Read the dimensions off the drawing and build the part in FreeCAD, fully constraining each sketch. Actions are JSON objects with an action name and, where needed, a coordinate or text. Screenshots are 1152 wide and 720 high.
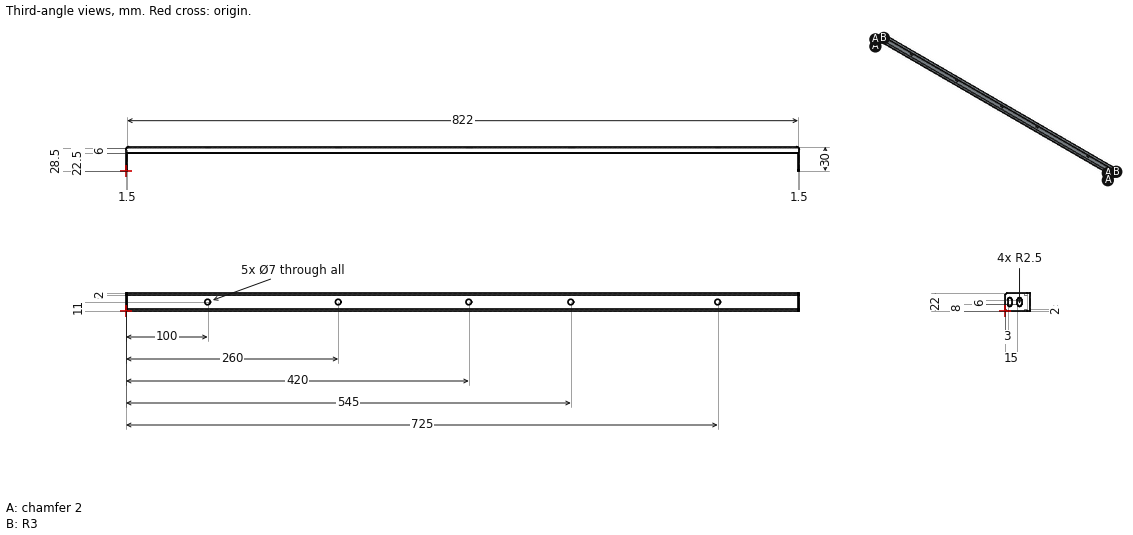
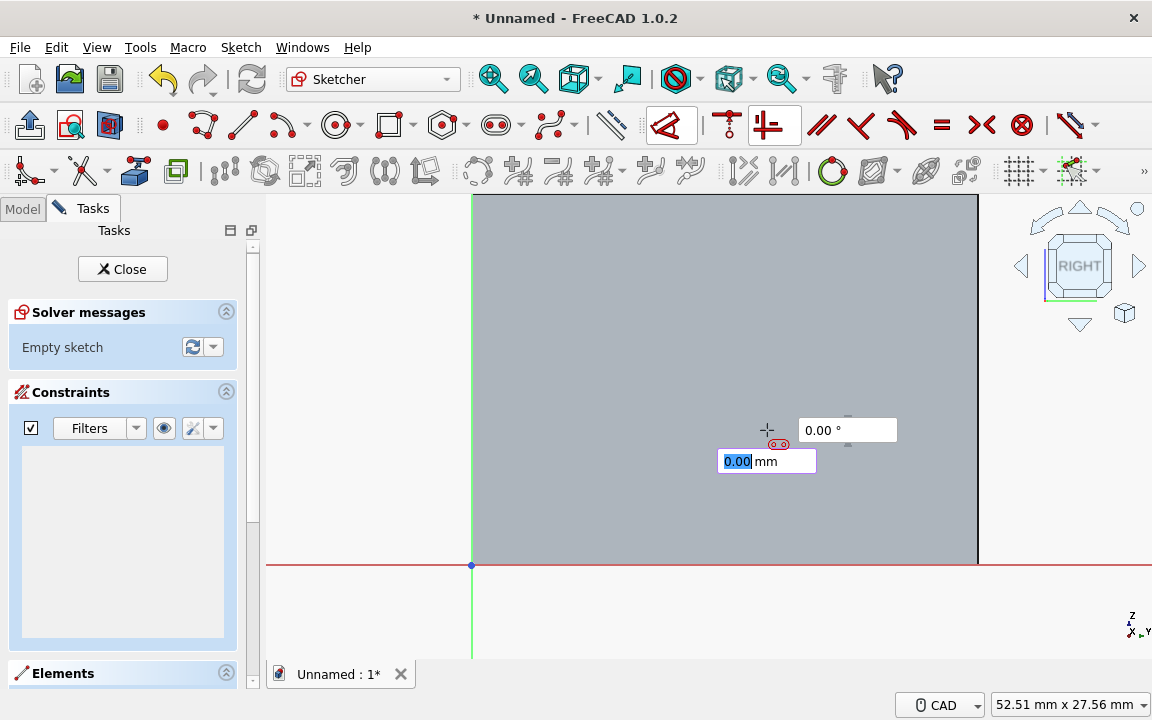
{"action": "left_click", "coordinate": [767, 329]}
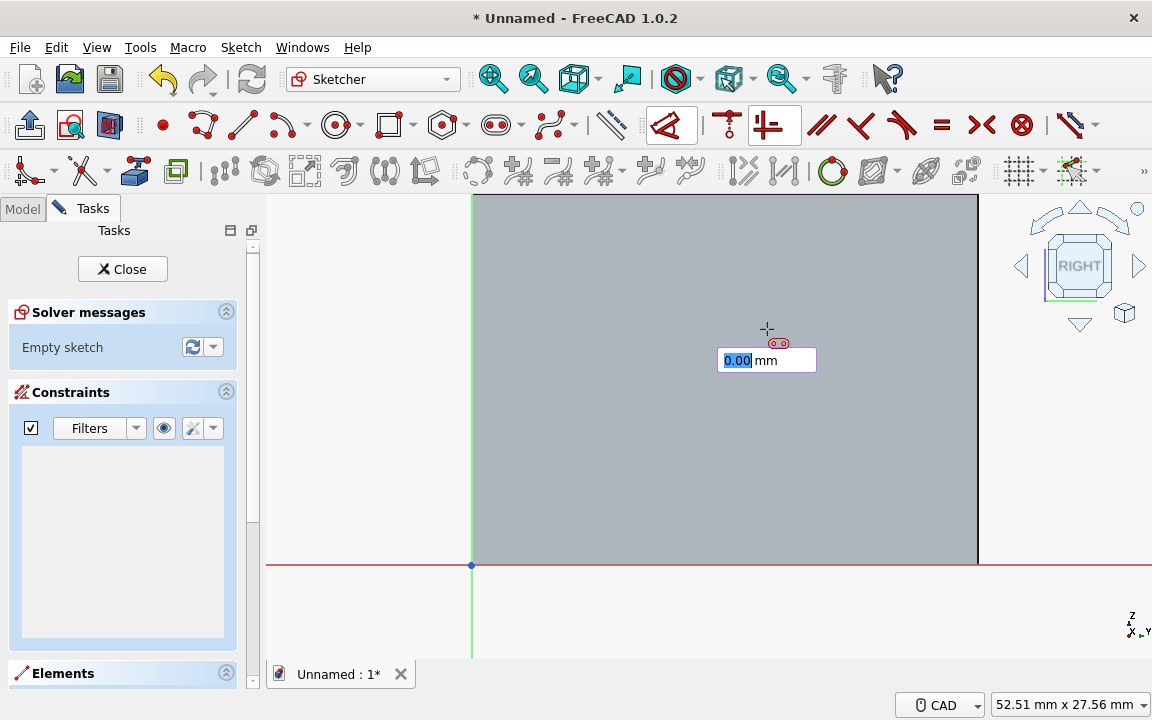
{"action": "left_click", "coordinate": [809, 380]}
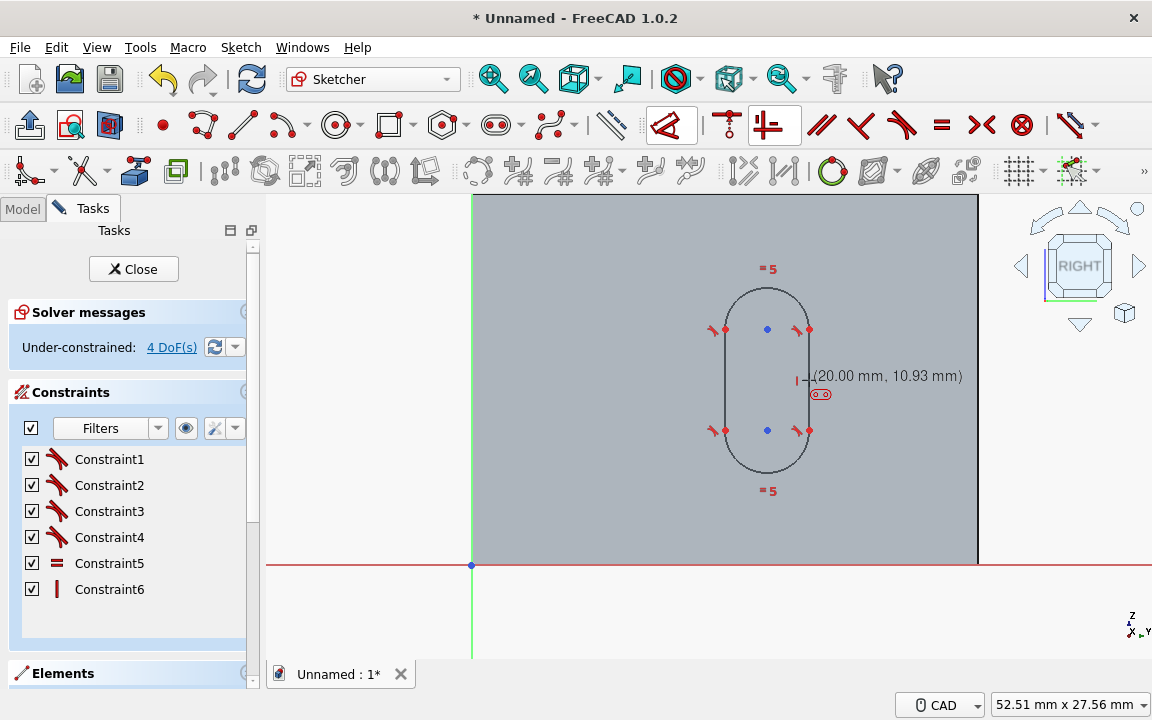
{"action": "left_click", "coordinate": [564, 430]}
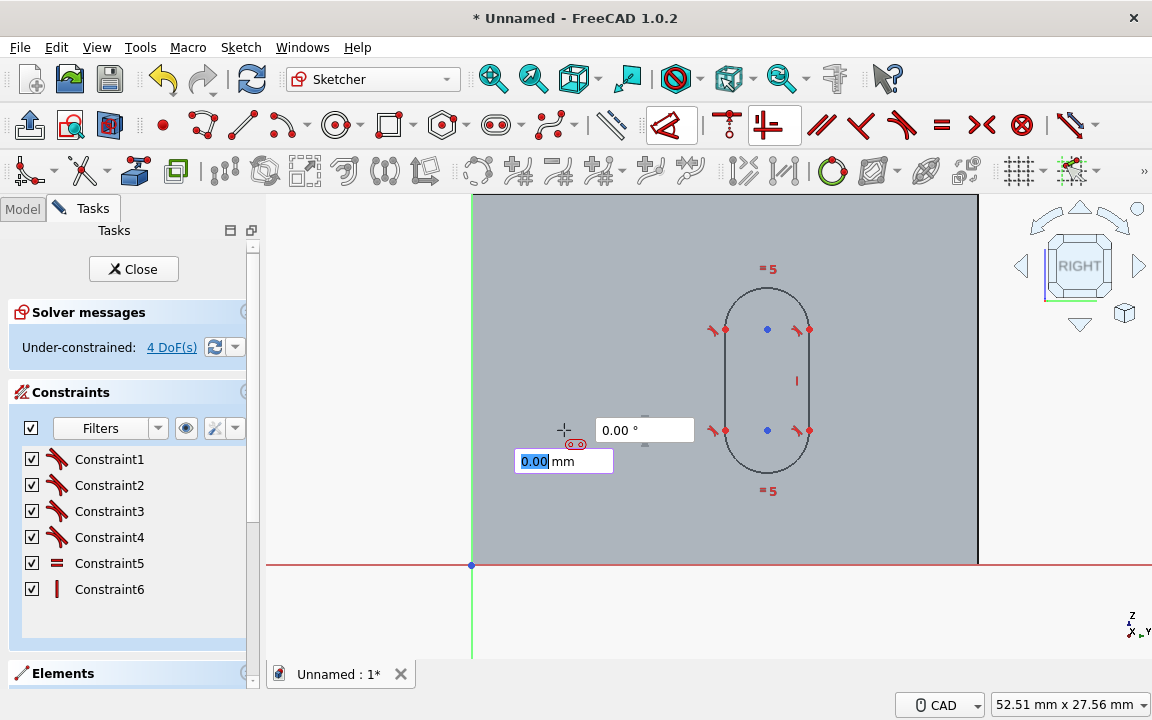
{"action": "left_click", "coordinate": [564, 329]}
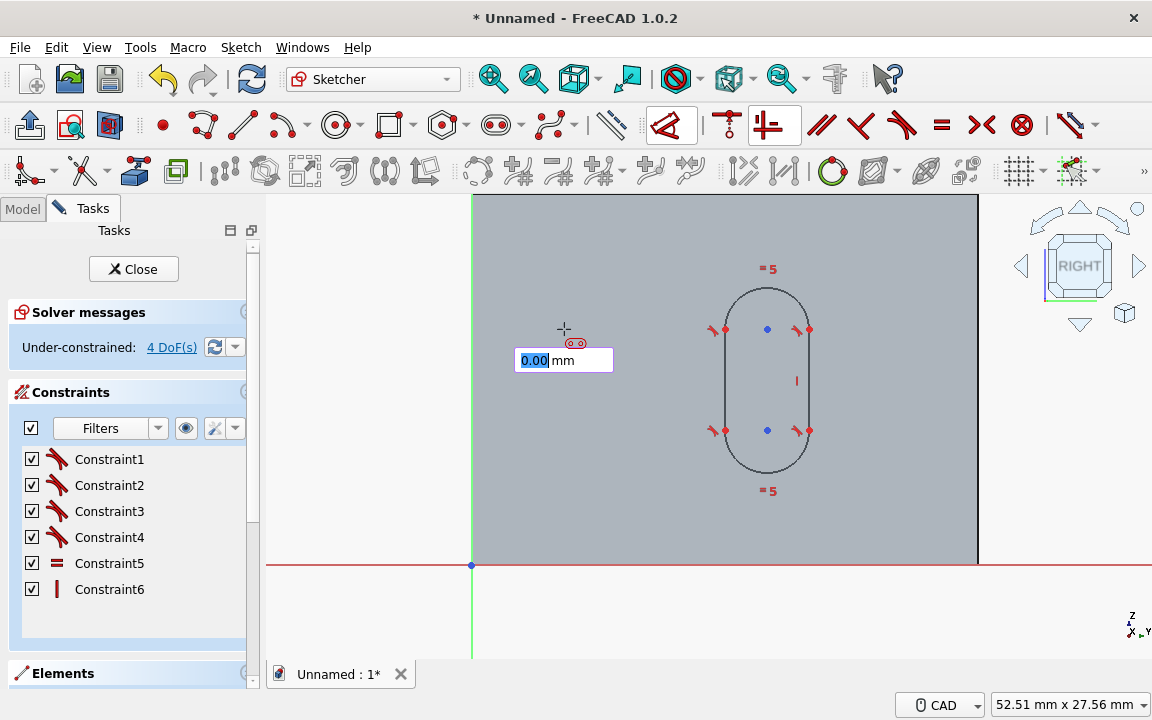
{"action": "left_click", "coordinate": [606, 380]}
{"action": "key", "text": "Escape"}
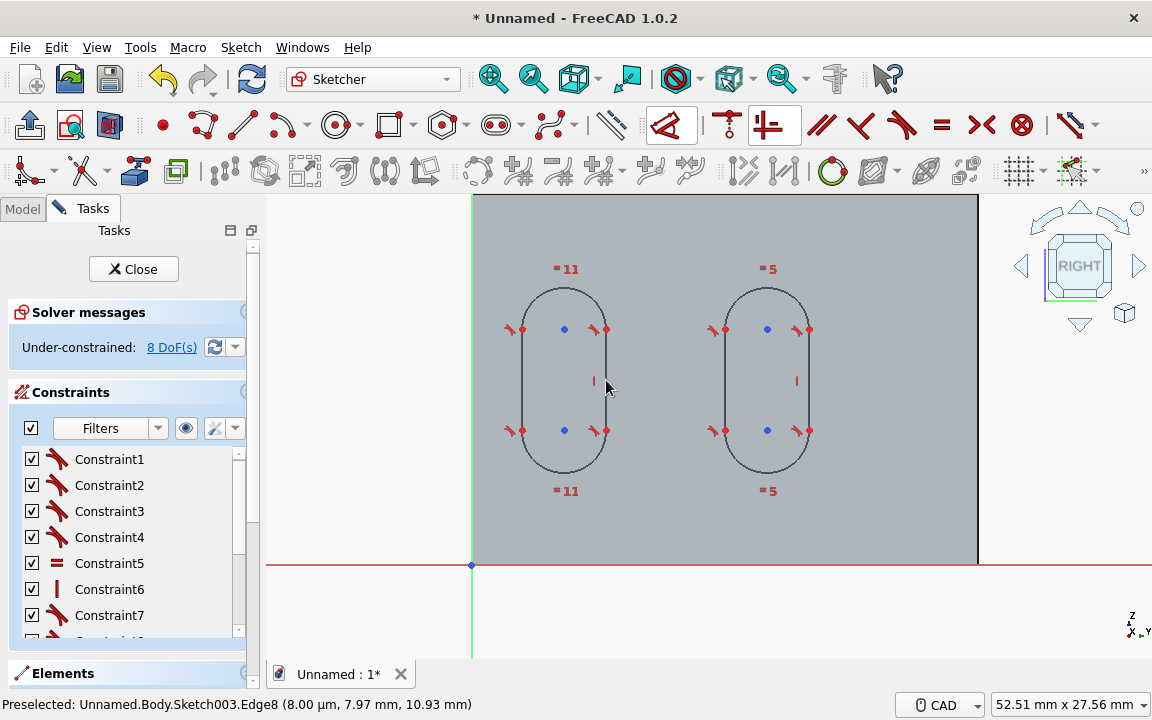
{"action": "left_click", "coordinate": [742, 465]}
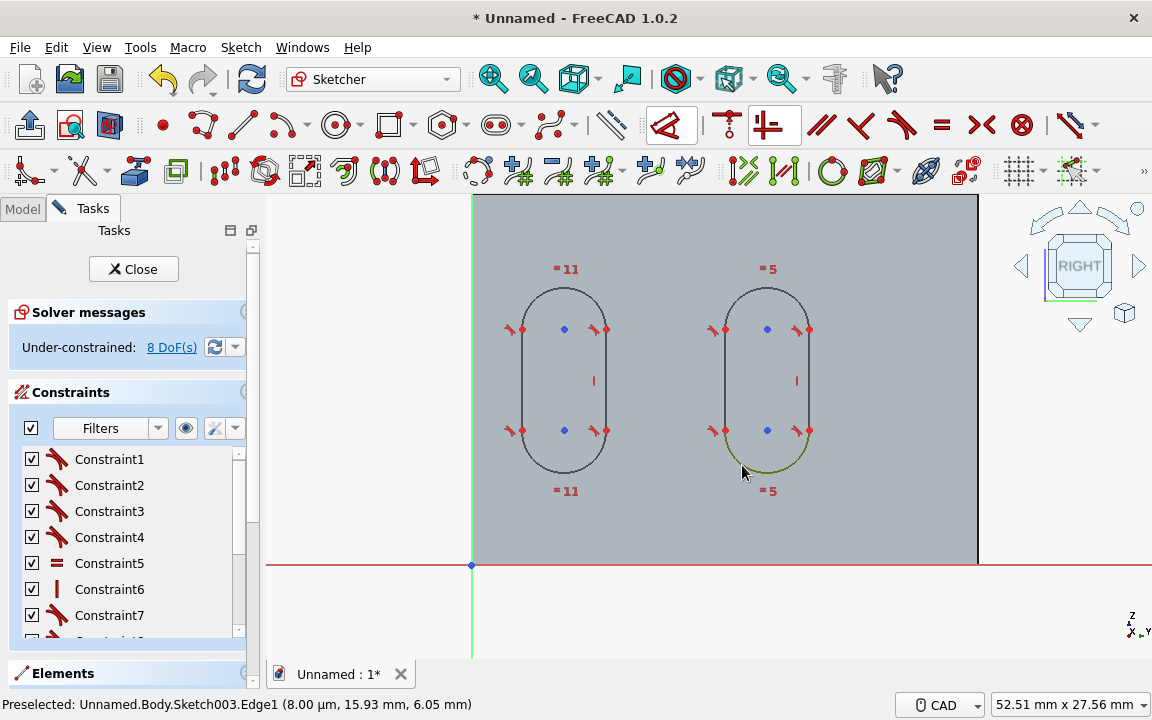
{"action": "left_click", "coordinate": [539, 465]}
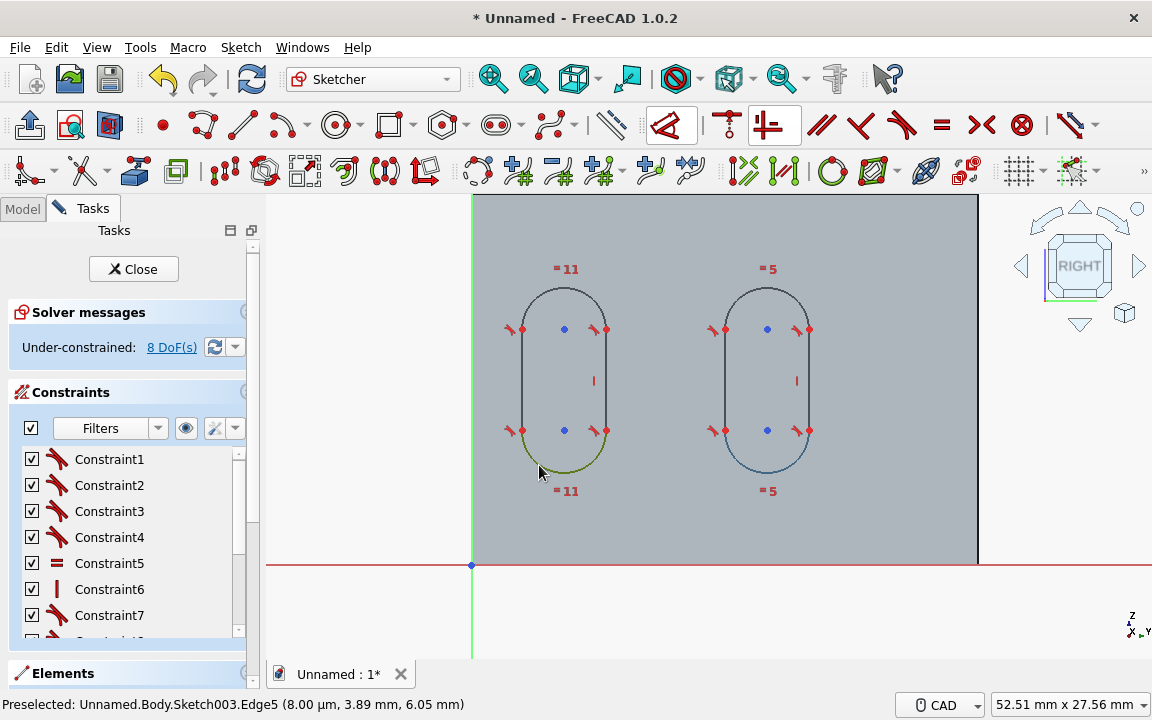
{"action": "left_click", "coordinate": [942, 126]}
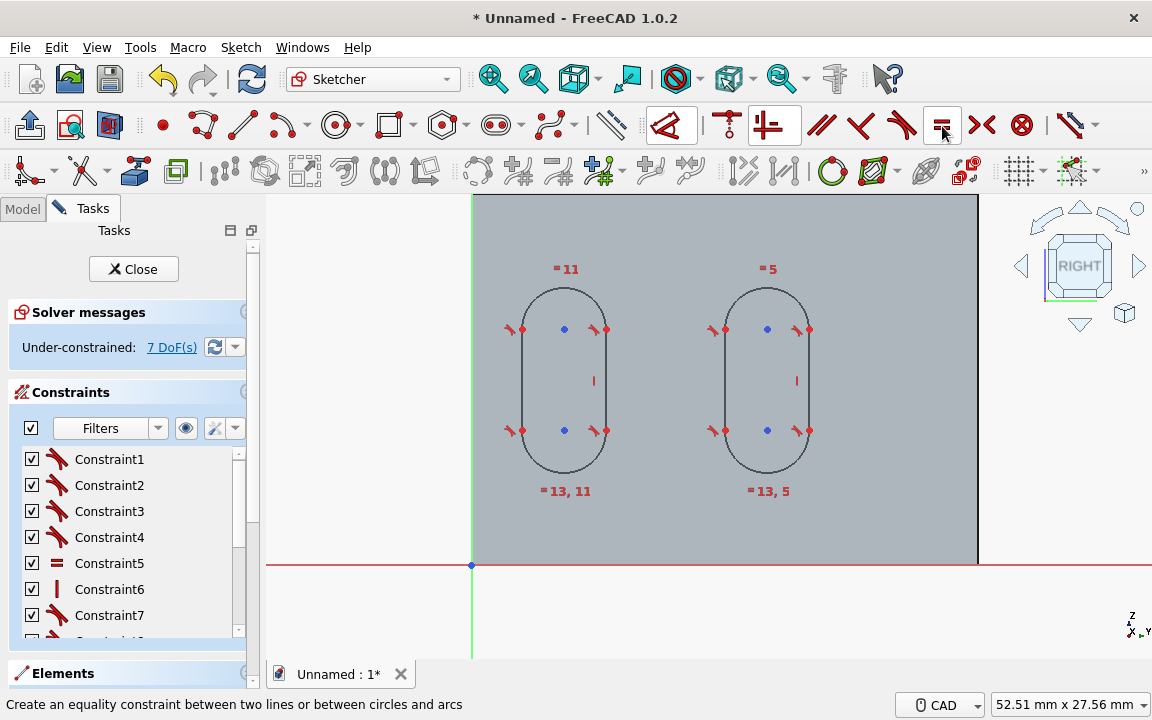
{"action": "left_click", "coordinate": [742, 465]}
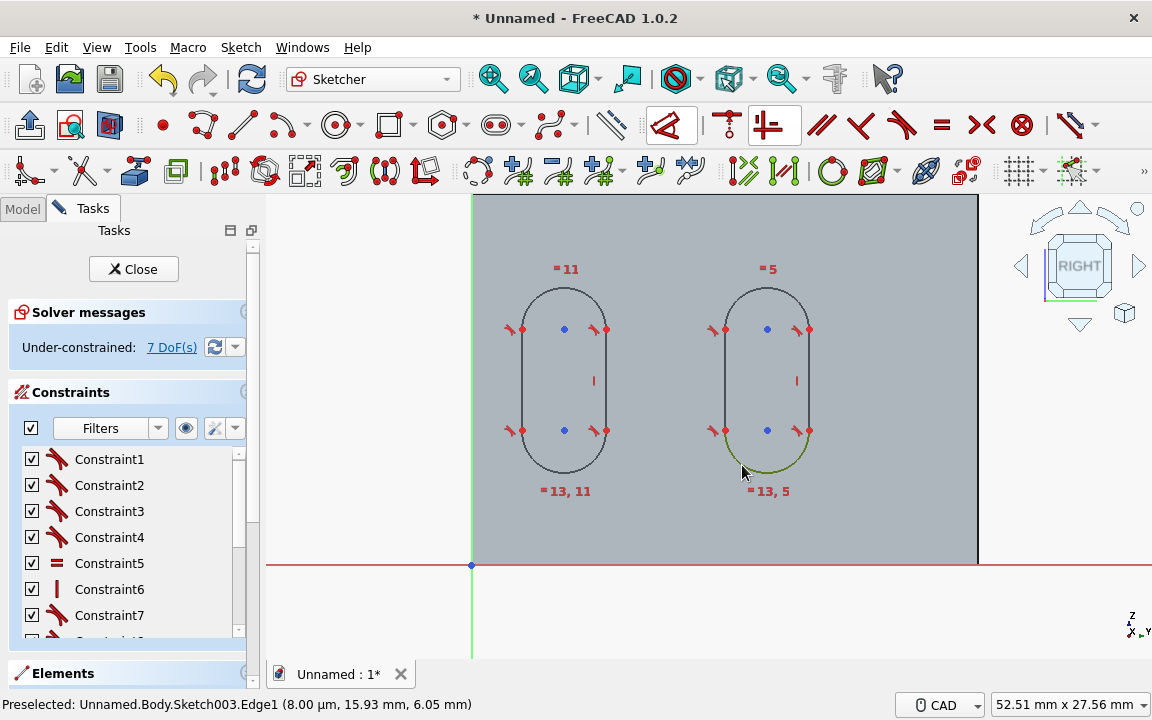
{"action": "left_click", "coordinate": [692, 126]}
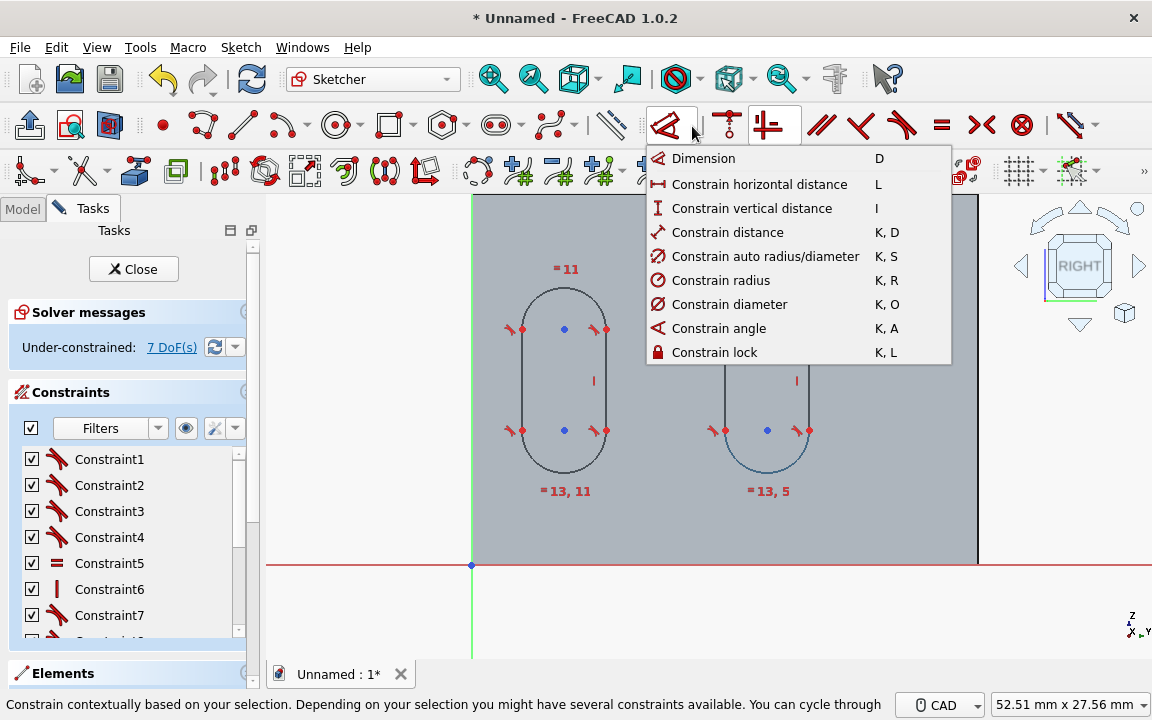
{"action": "left_click", "coordinate": [799, 280]}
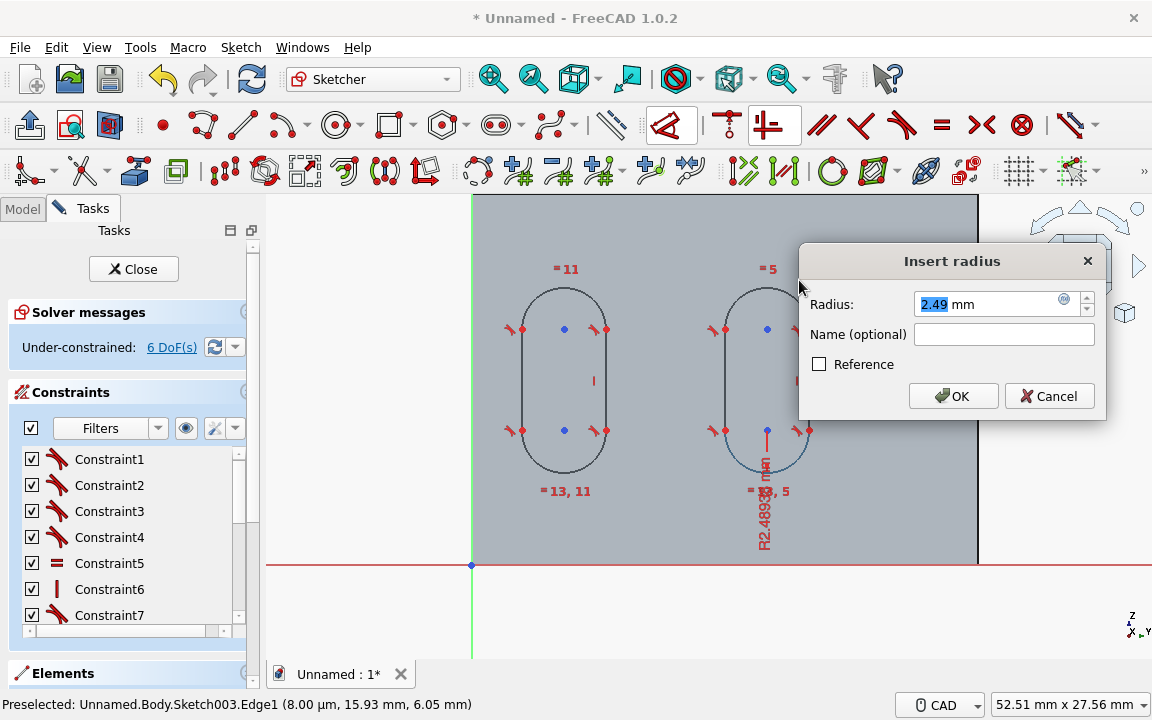
{"action": "type", "text": "2.5"}
{"action": "key", "text": "Return"}